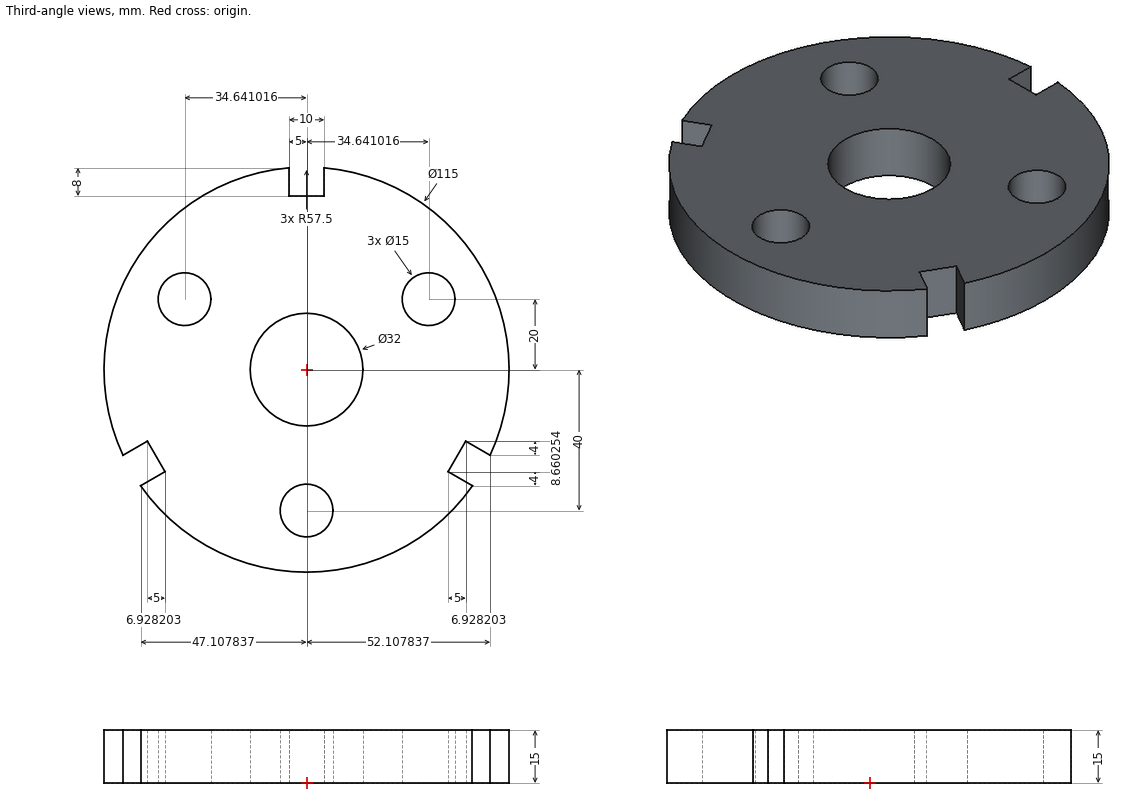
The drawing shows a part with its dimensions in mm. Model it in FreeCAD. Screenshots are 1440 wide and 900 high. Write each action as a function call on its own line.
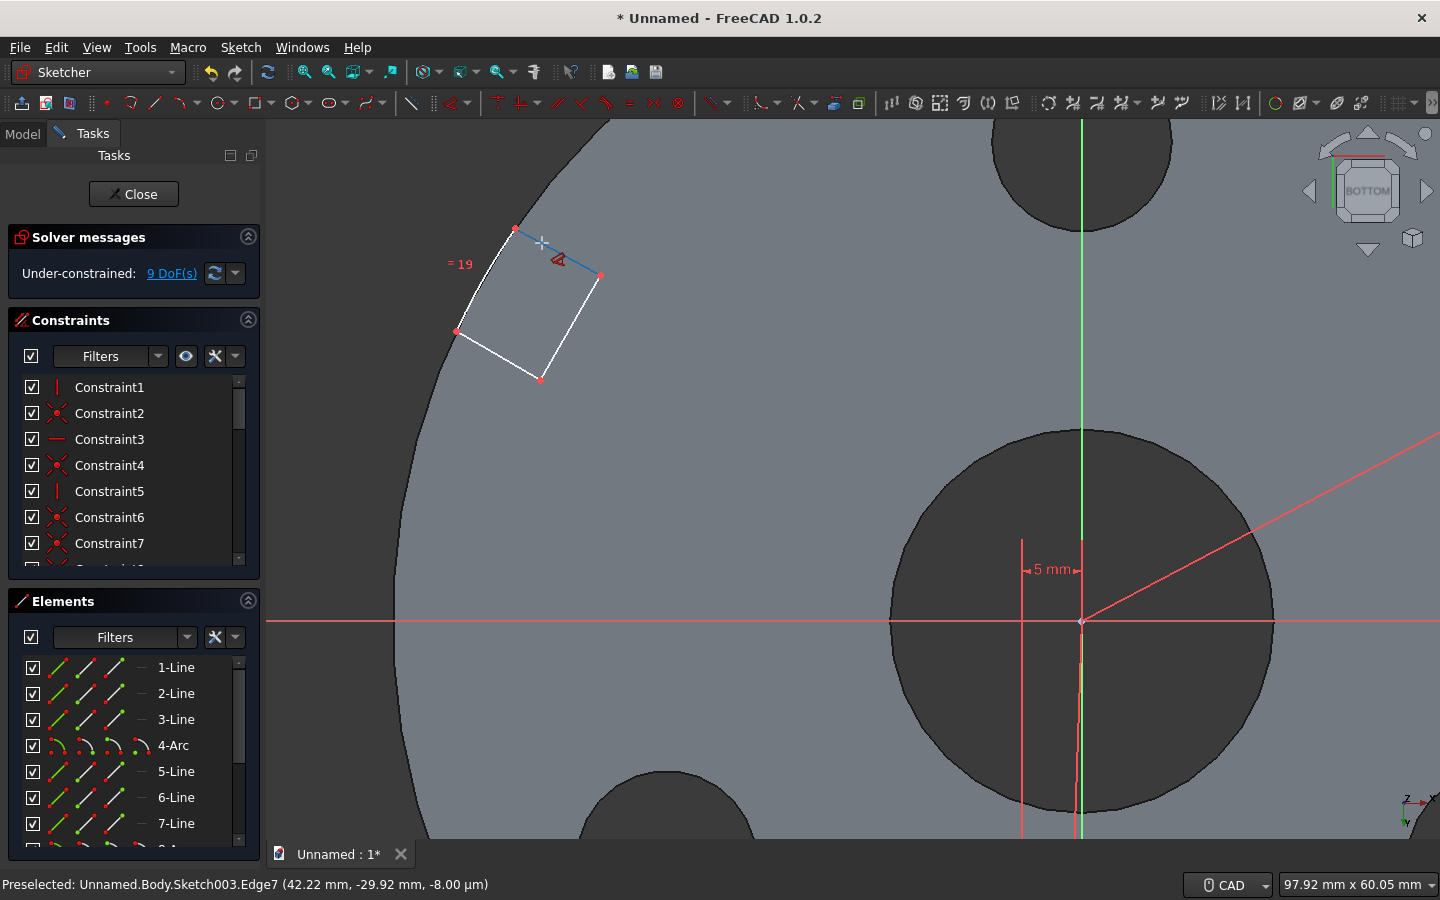
click(541, 243)
click(481, 252)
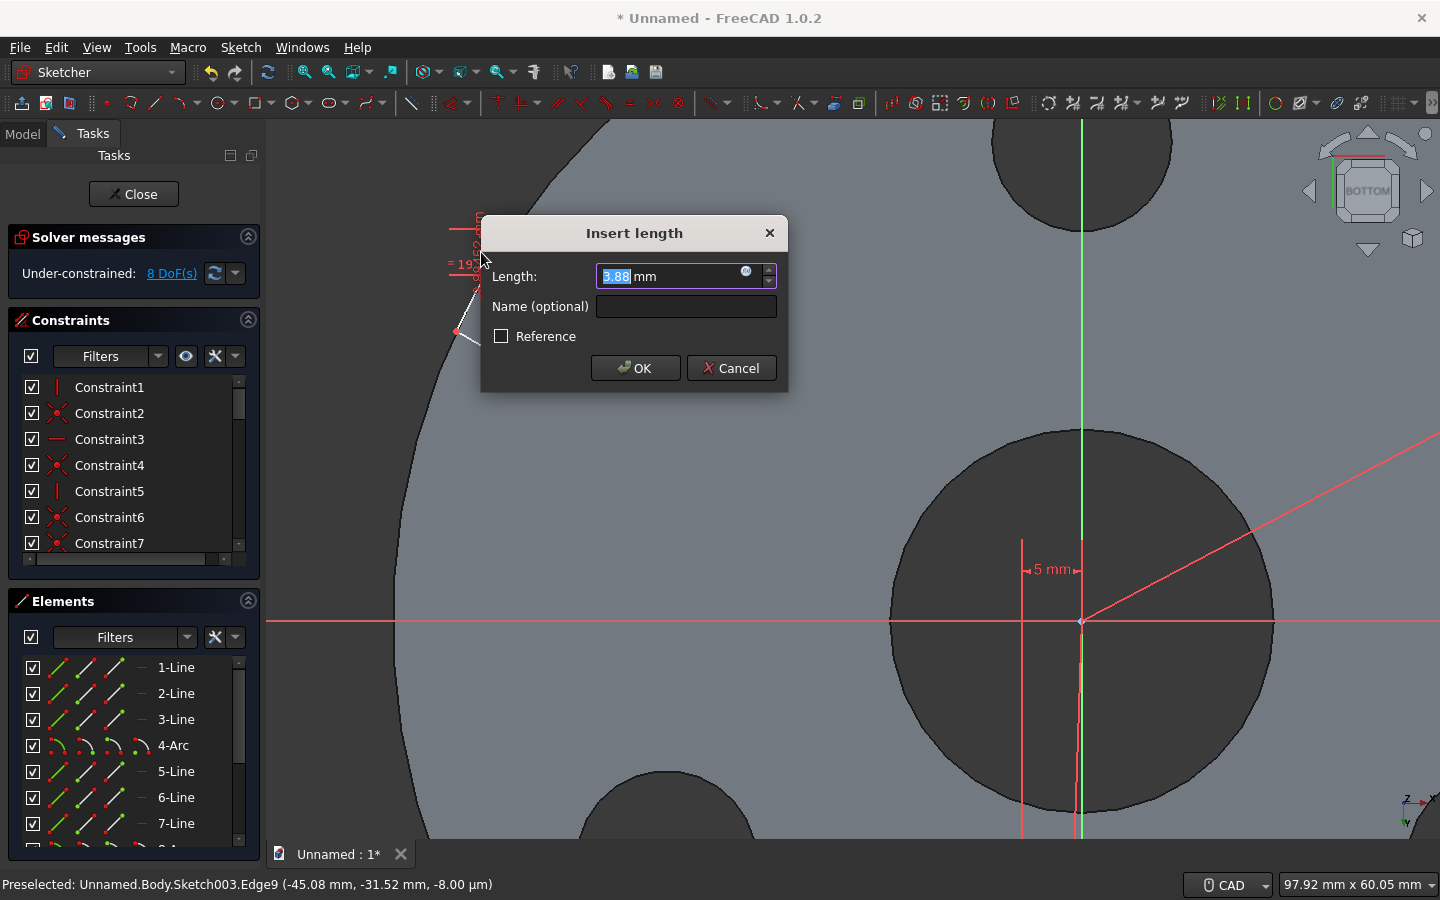
text(4)
key(Return)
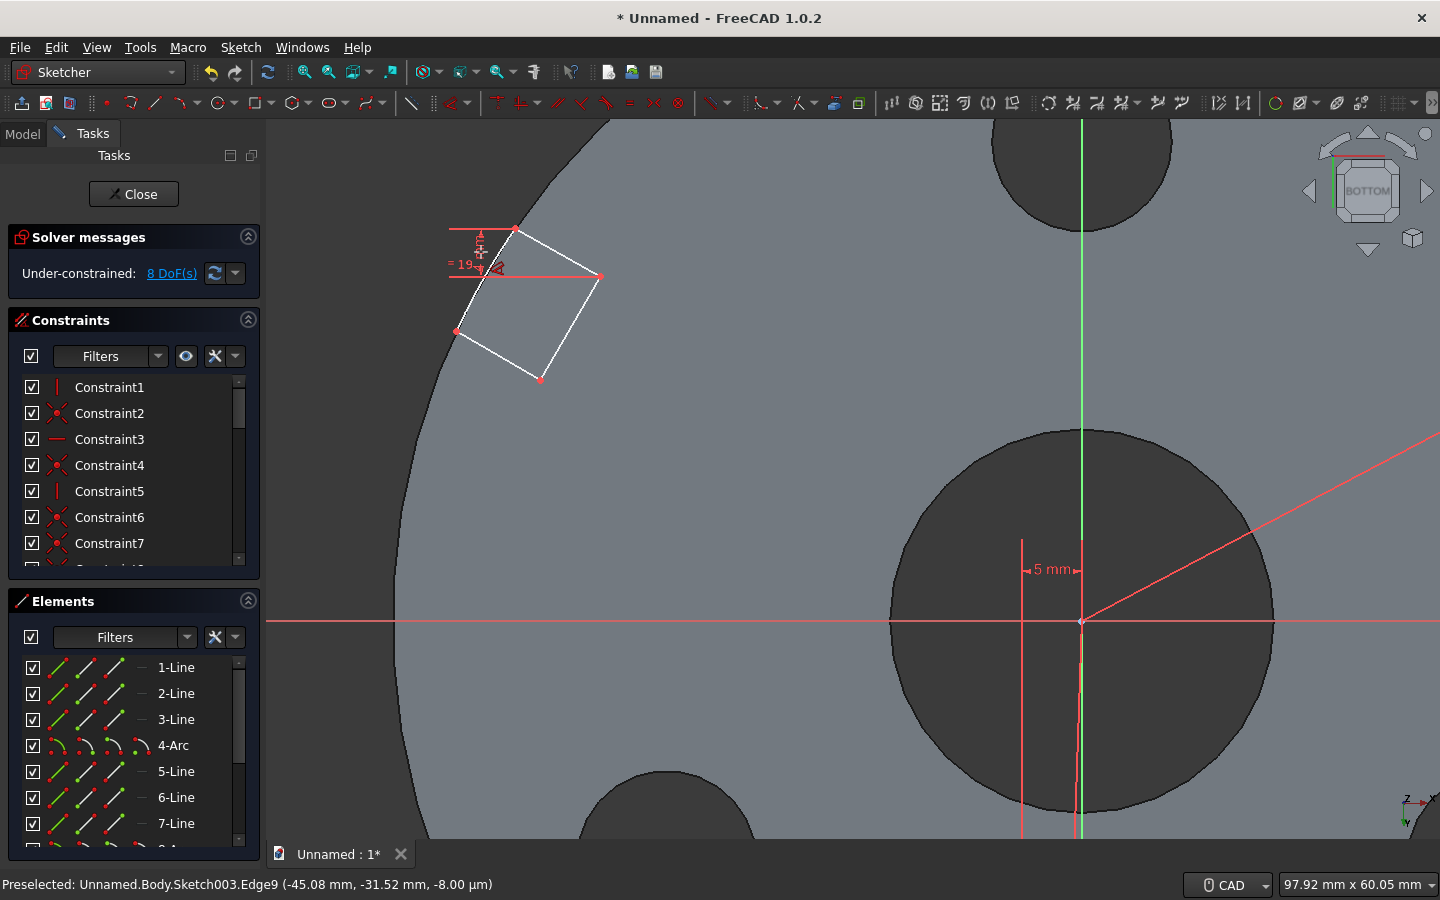
click(582, 308)
click(570, 243)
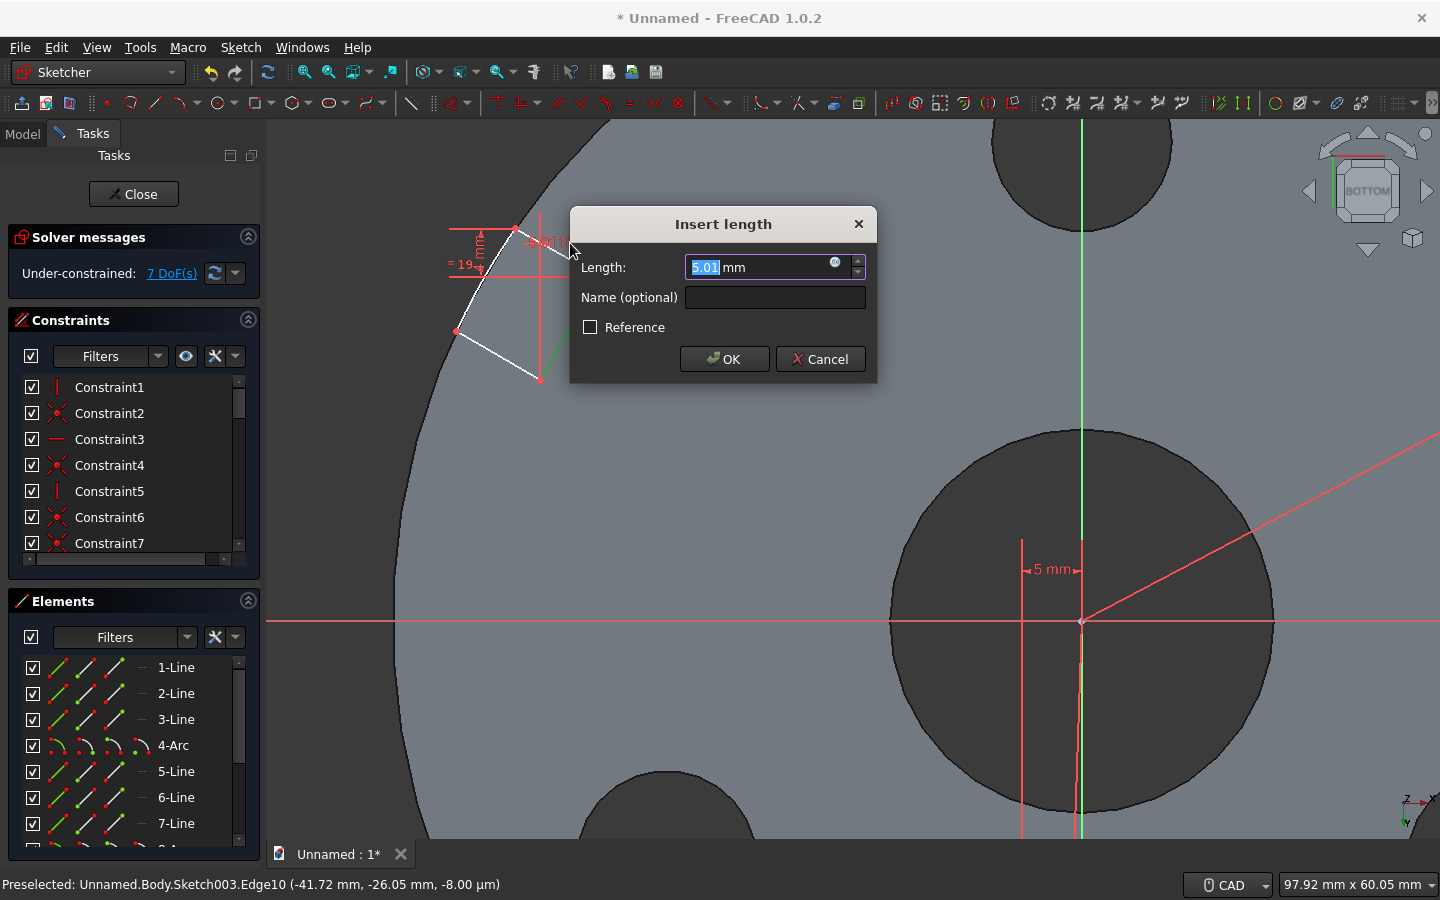
text(5)
key(Return)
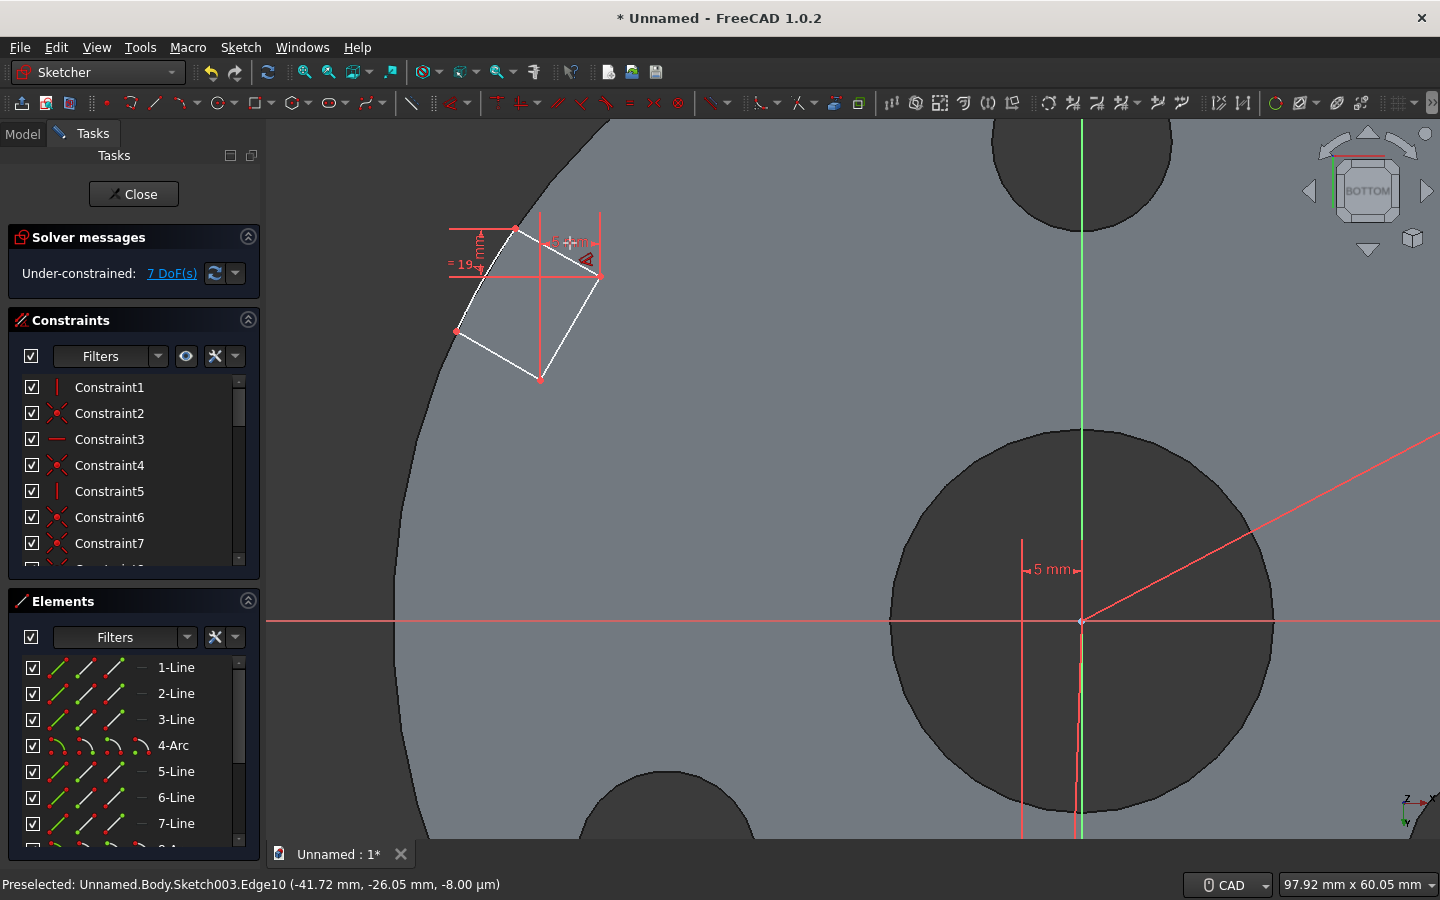
click(515, 365)
click(422, 356)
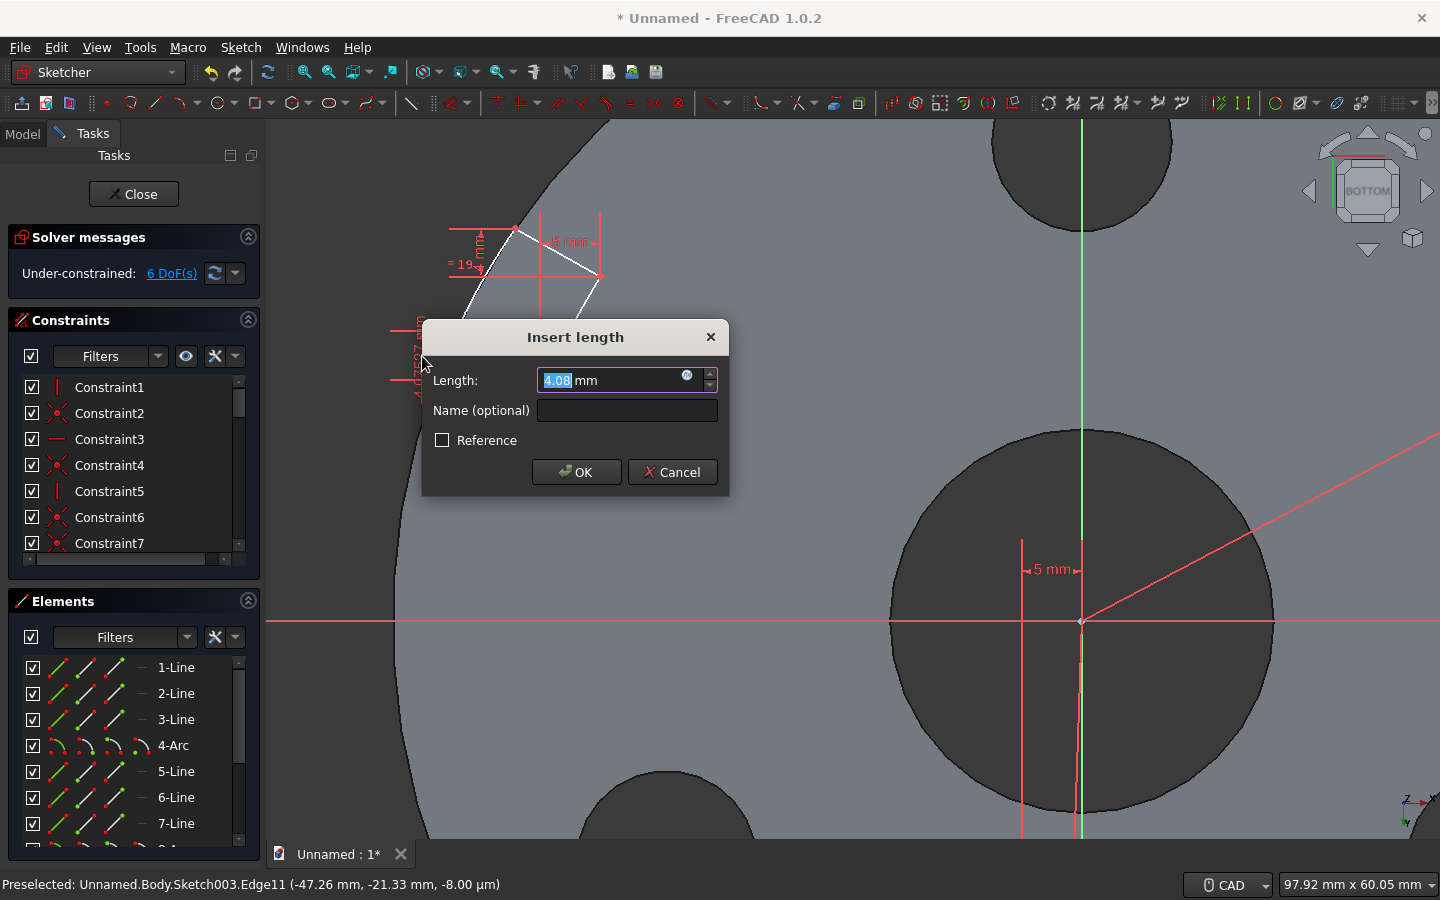
text(4)
key(Return)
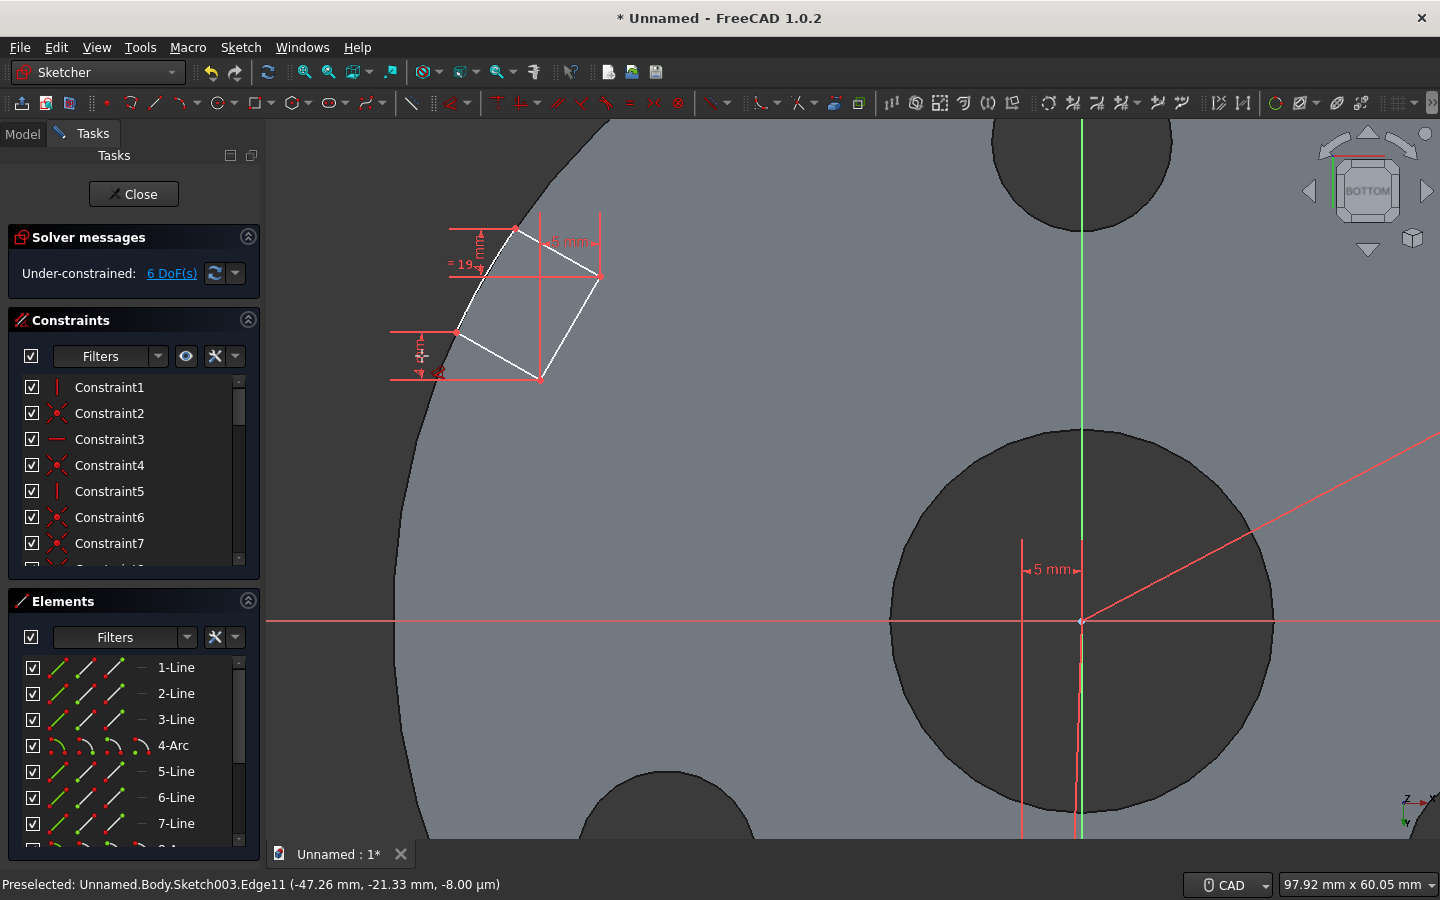
scroll(542, 243, down, 4)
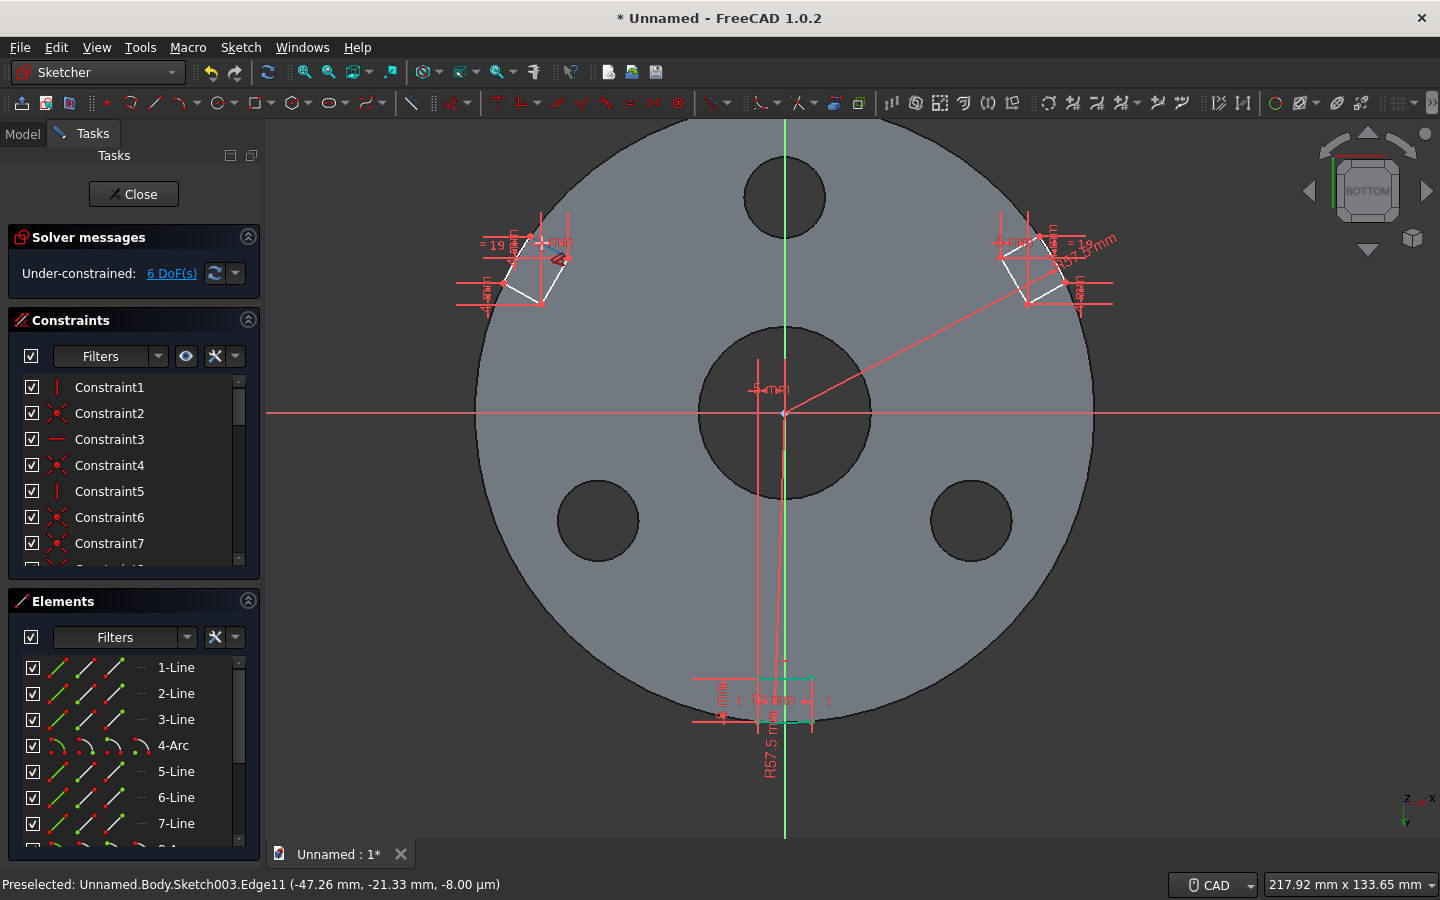
click(1054, 289)
click(1047, 338)